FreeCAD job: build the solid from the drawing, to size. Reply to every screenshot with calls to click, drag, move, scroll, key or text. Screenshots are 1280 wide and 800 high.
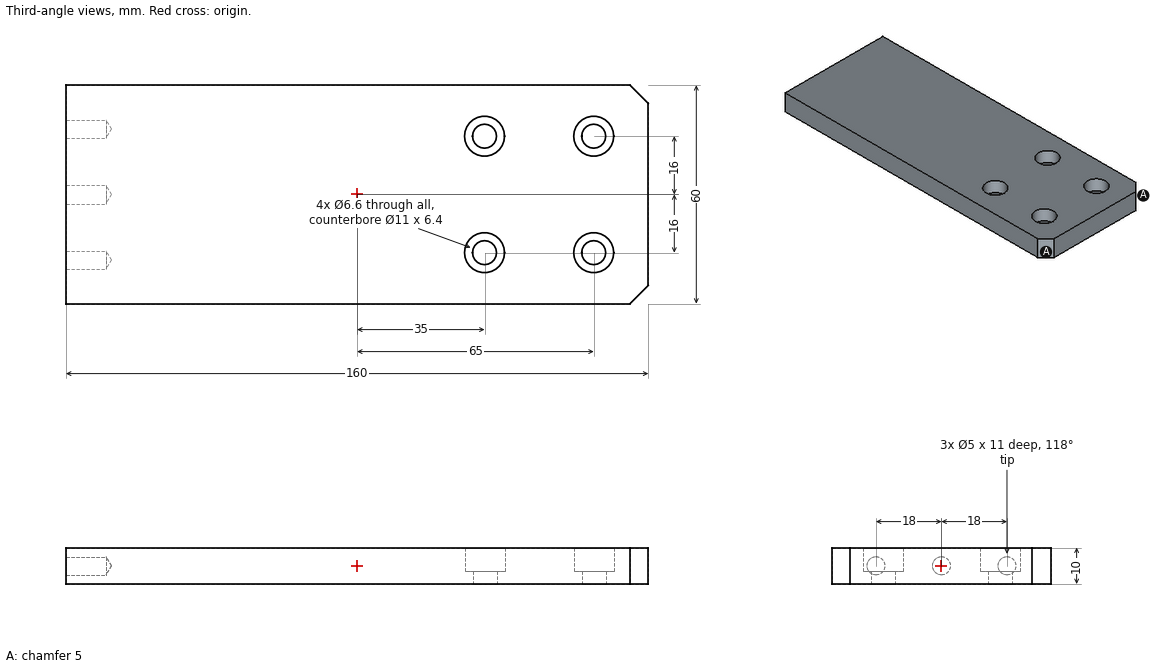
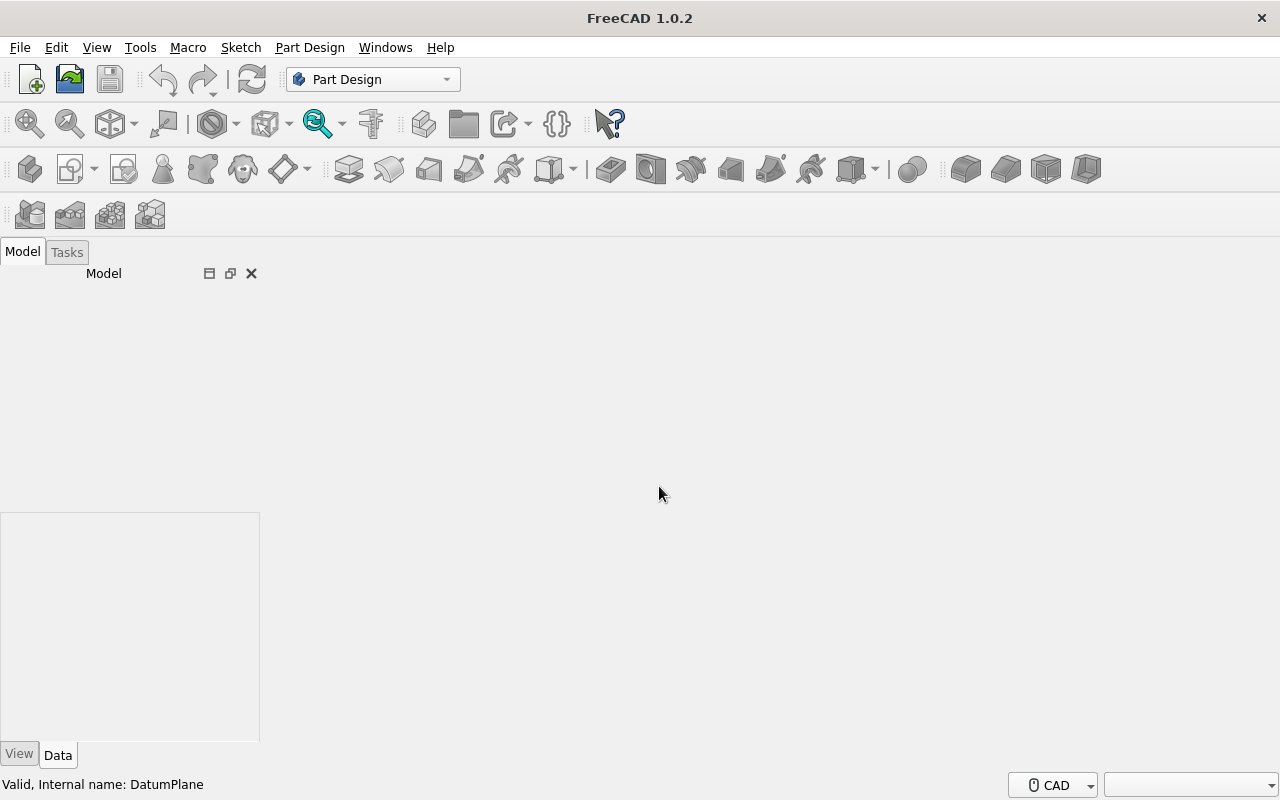
click(30, 80)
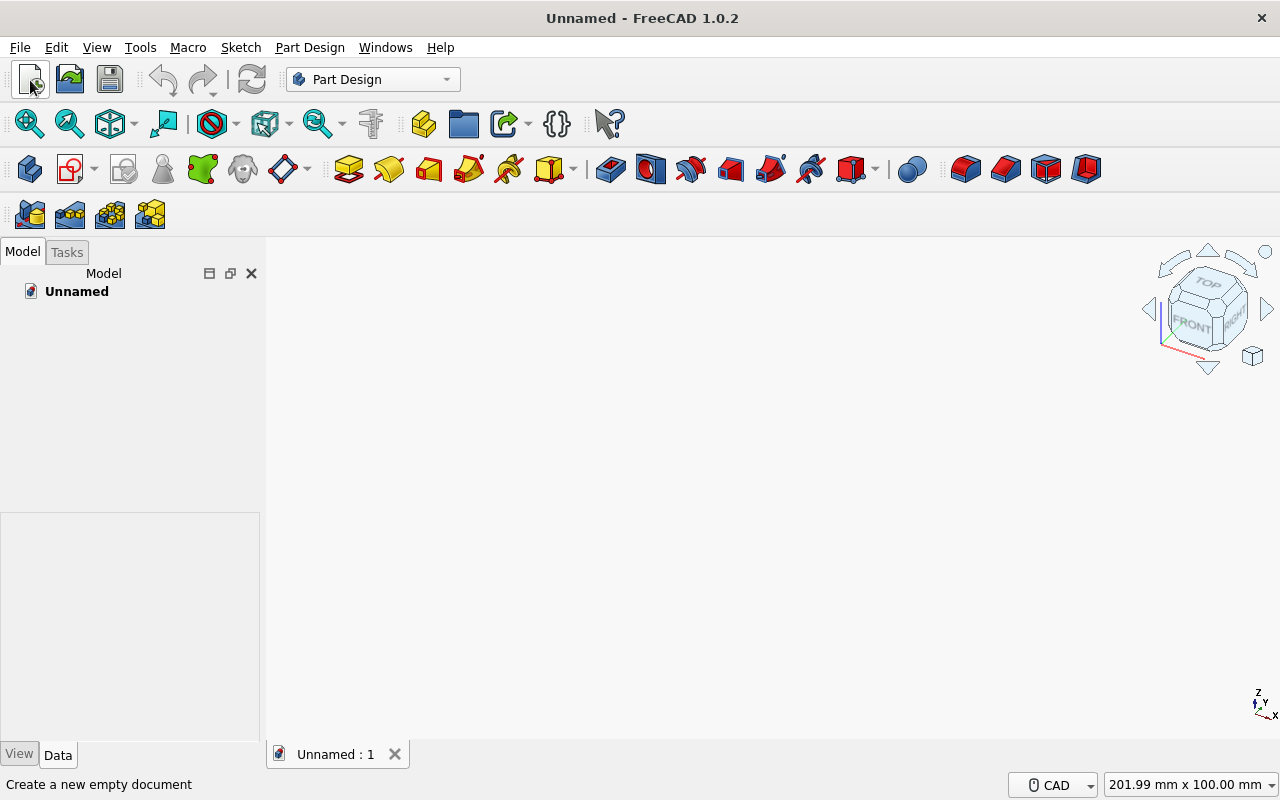
click(70, 170)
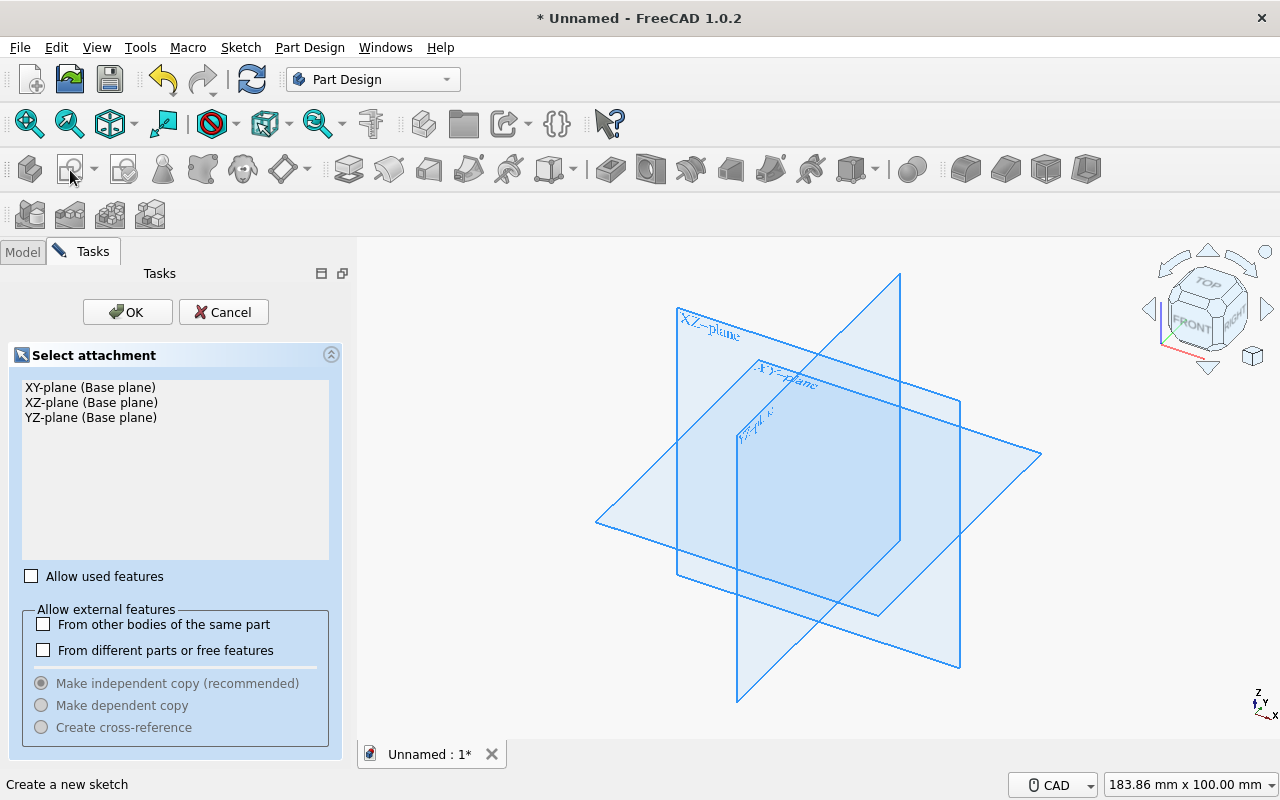
click(82, 388)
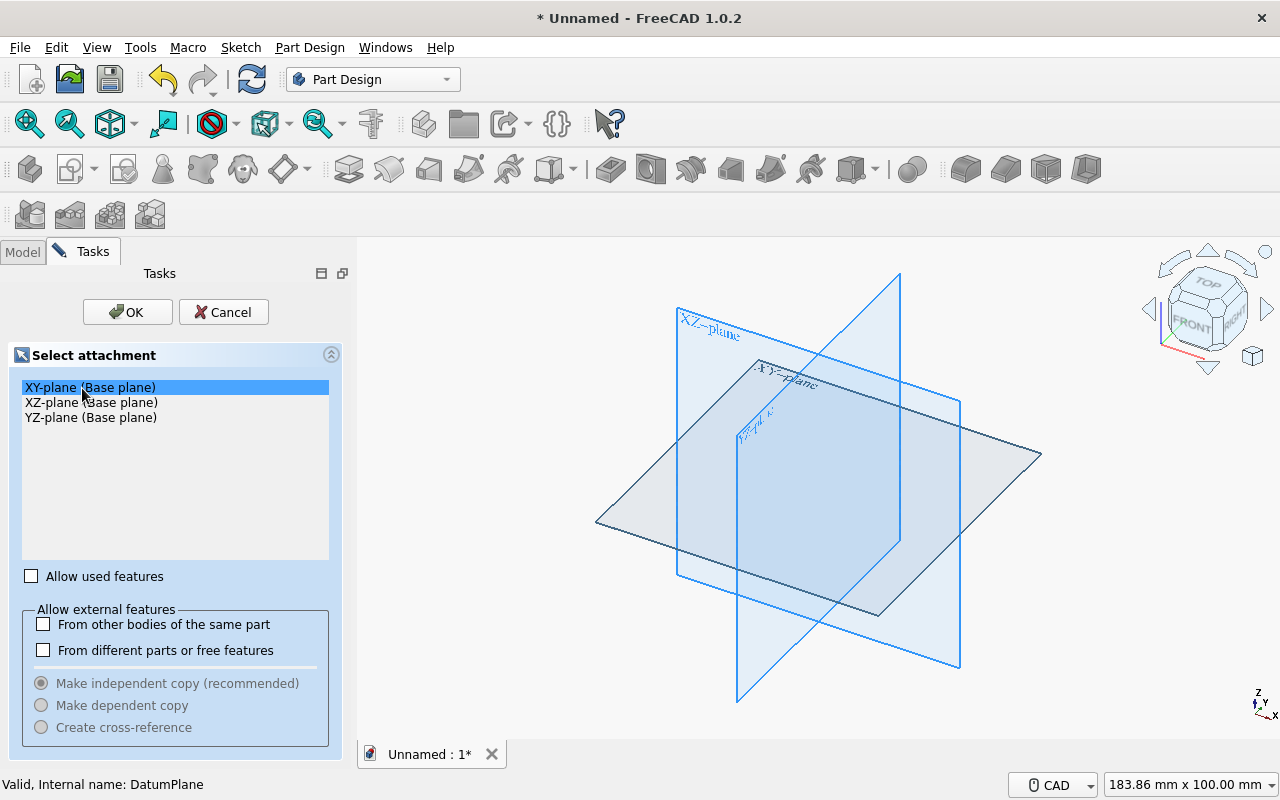
click(128, 312)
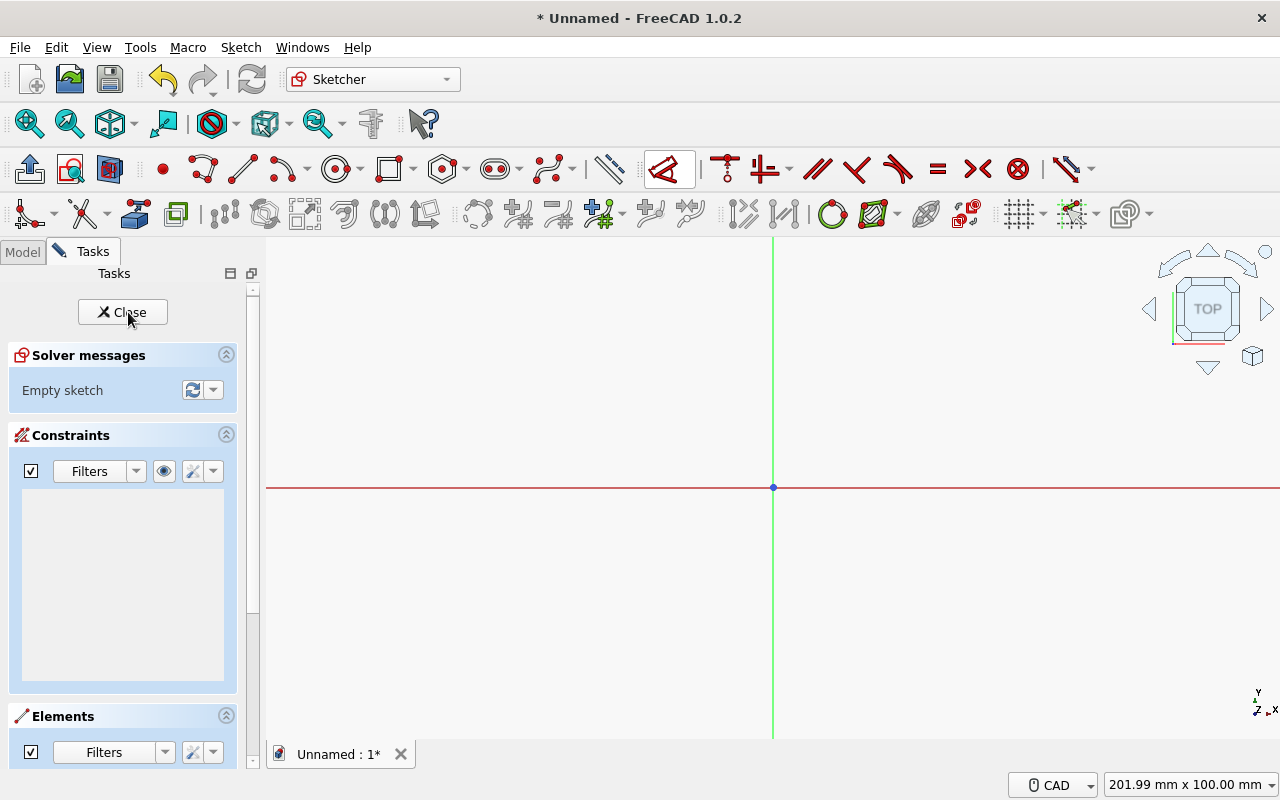
scroll(565, 488, down, 2)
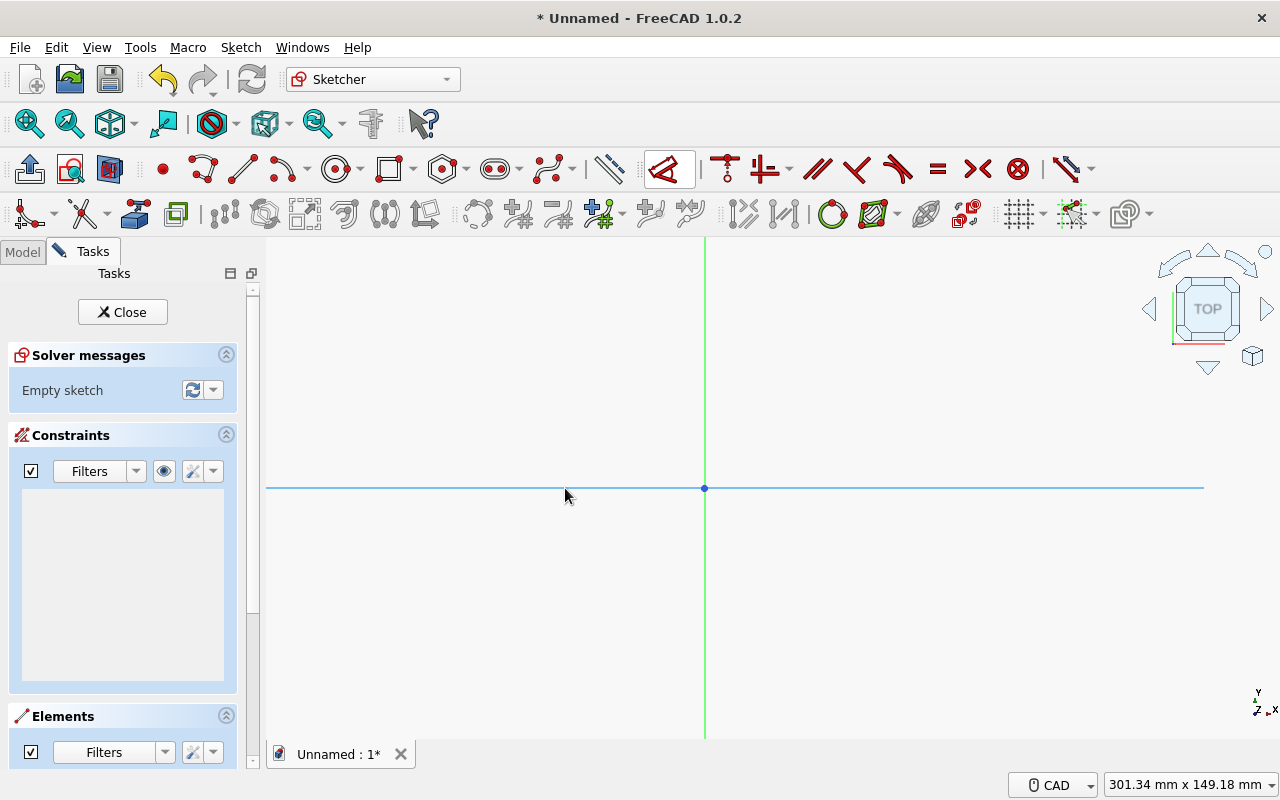
key(g)
key(v)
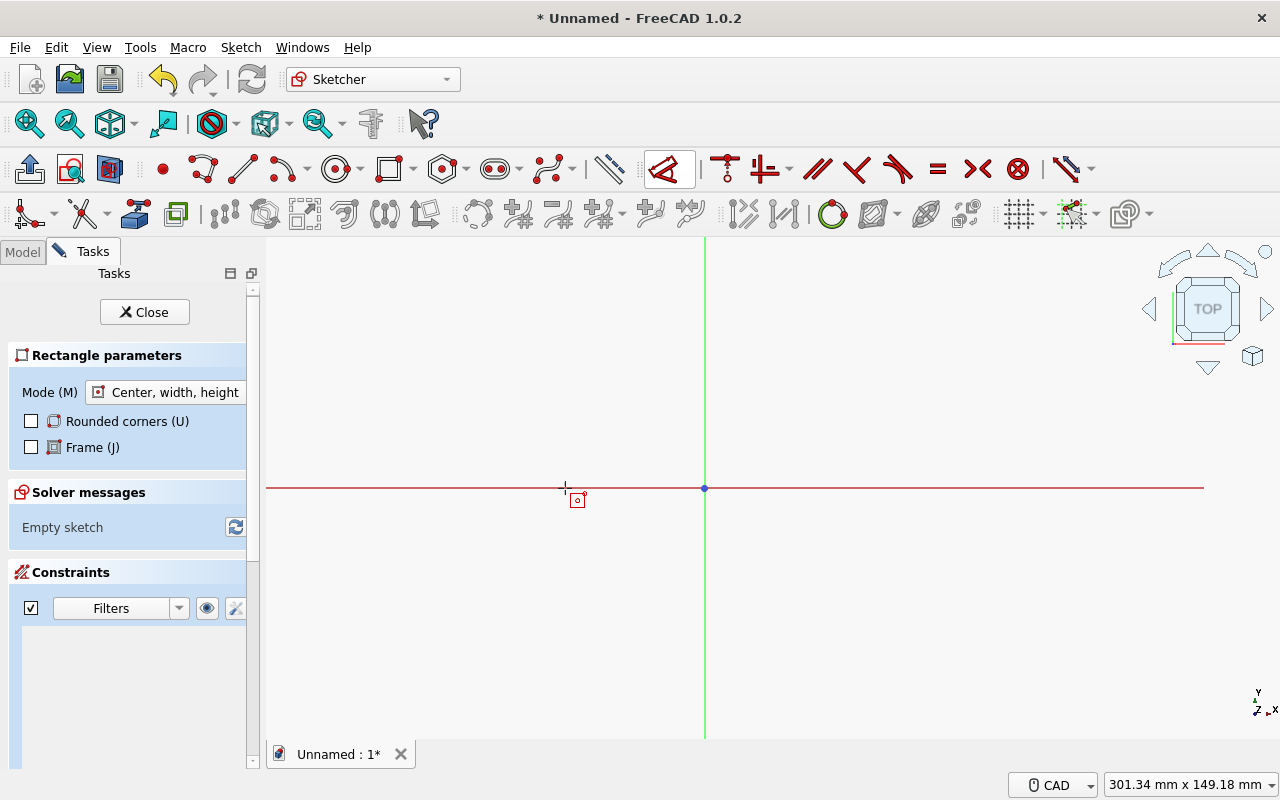
click(705, 488)
move(974, 387)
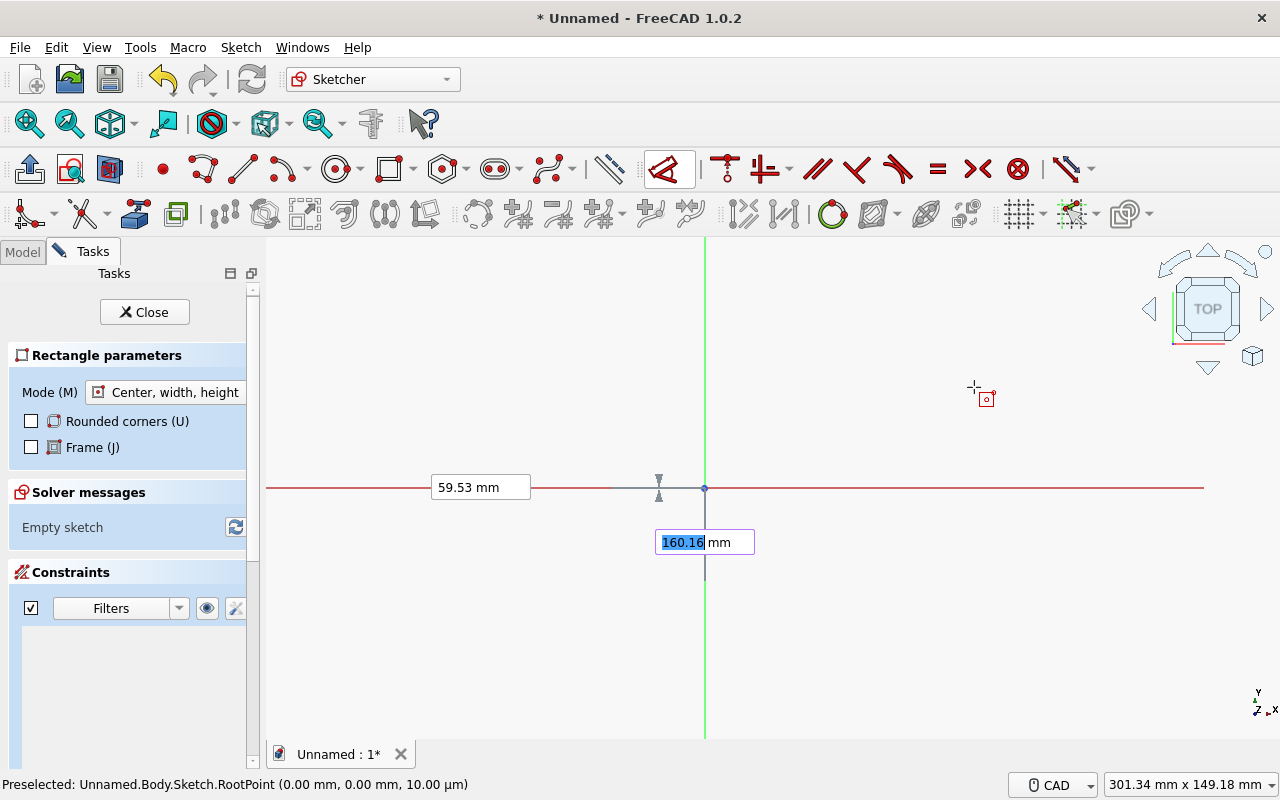
text(160)
key(Tab)
text(60)
key(Return)
key(Escape)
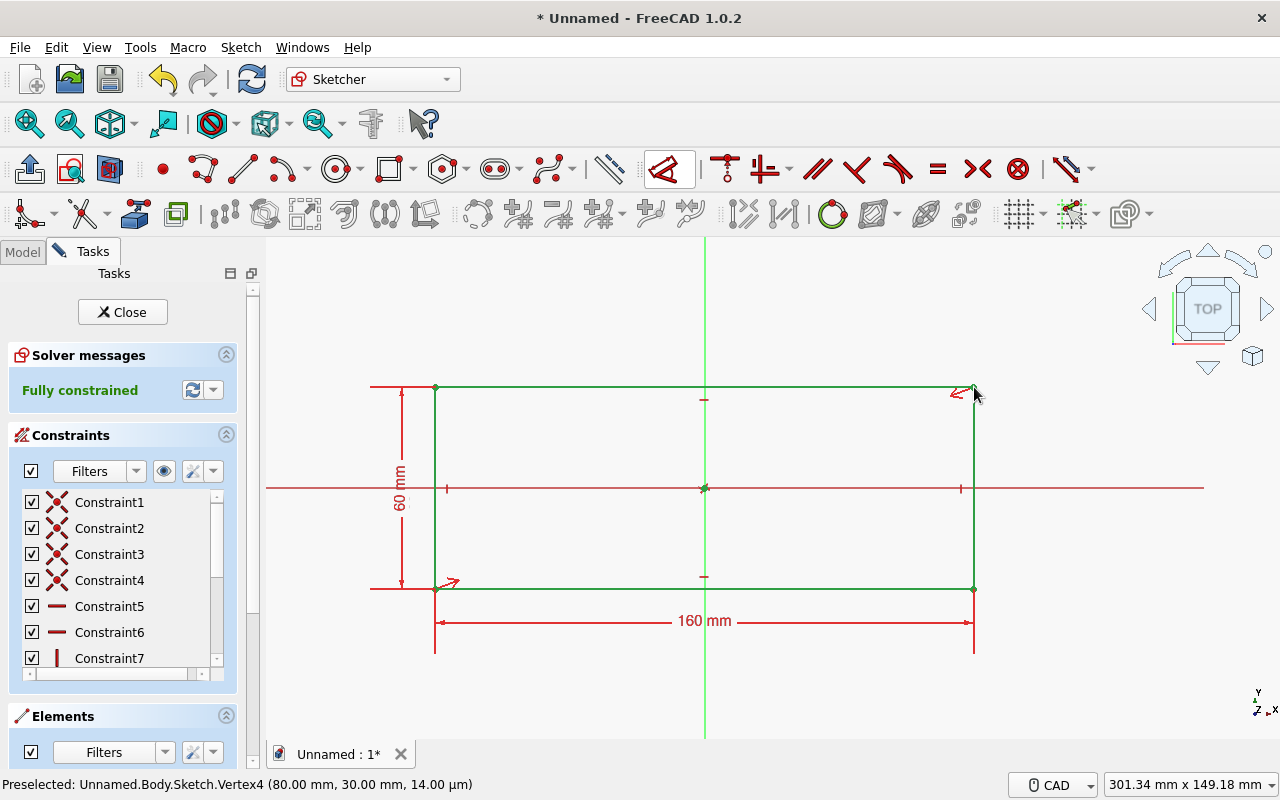
click(123, 312)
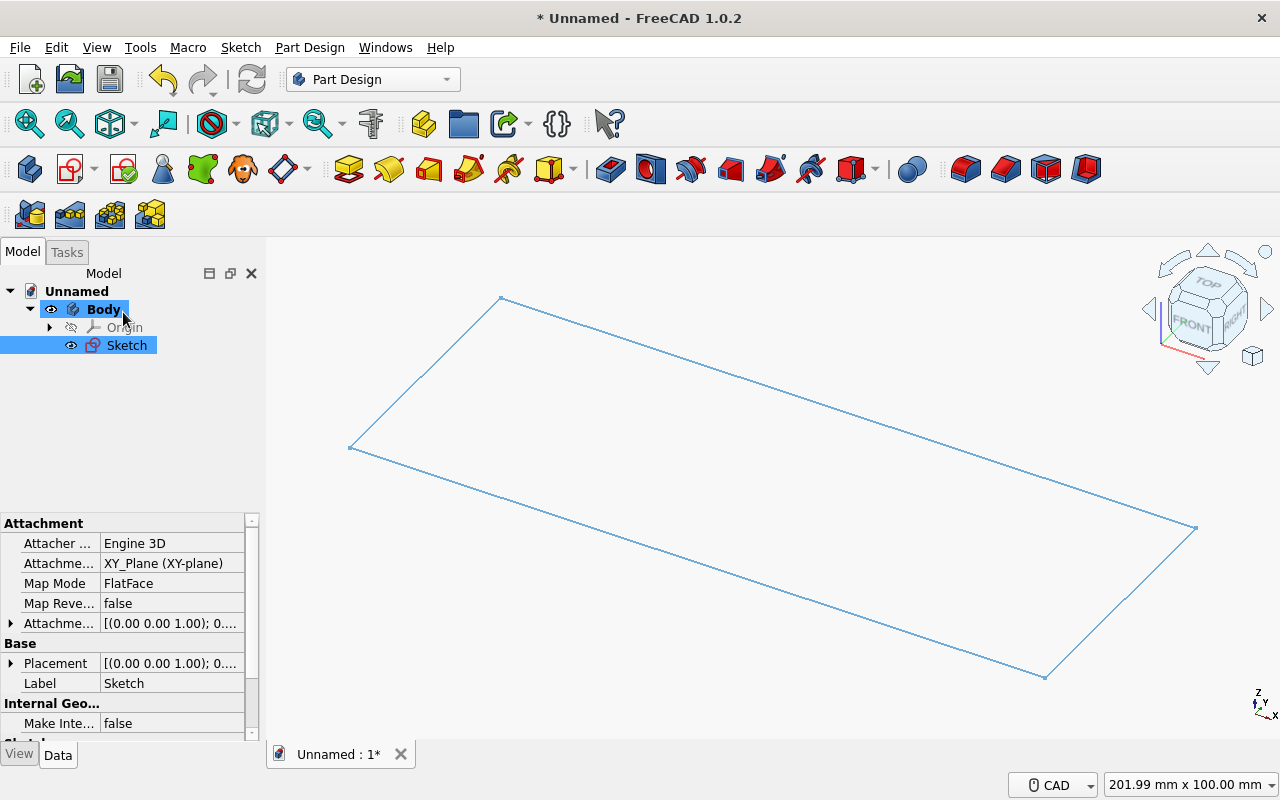
click(350, 170)